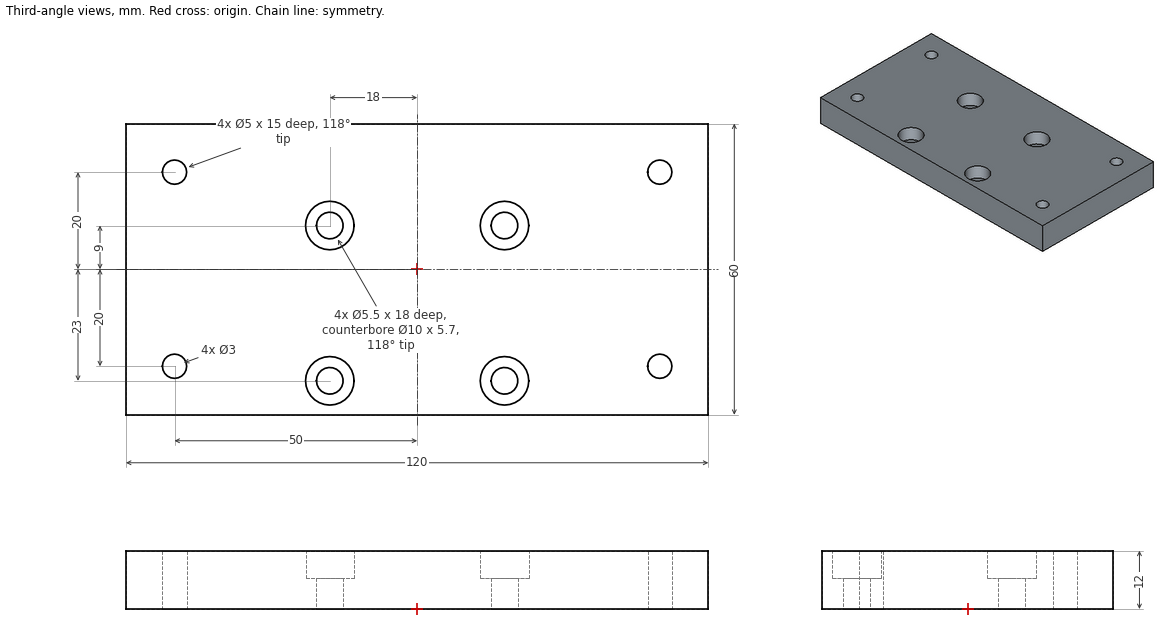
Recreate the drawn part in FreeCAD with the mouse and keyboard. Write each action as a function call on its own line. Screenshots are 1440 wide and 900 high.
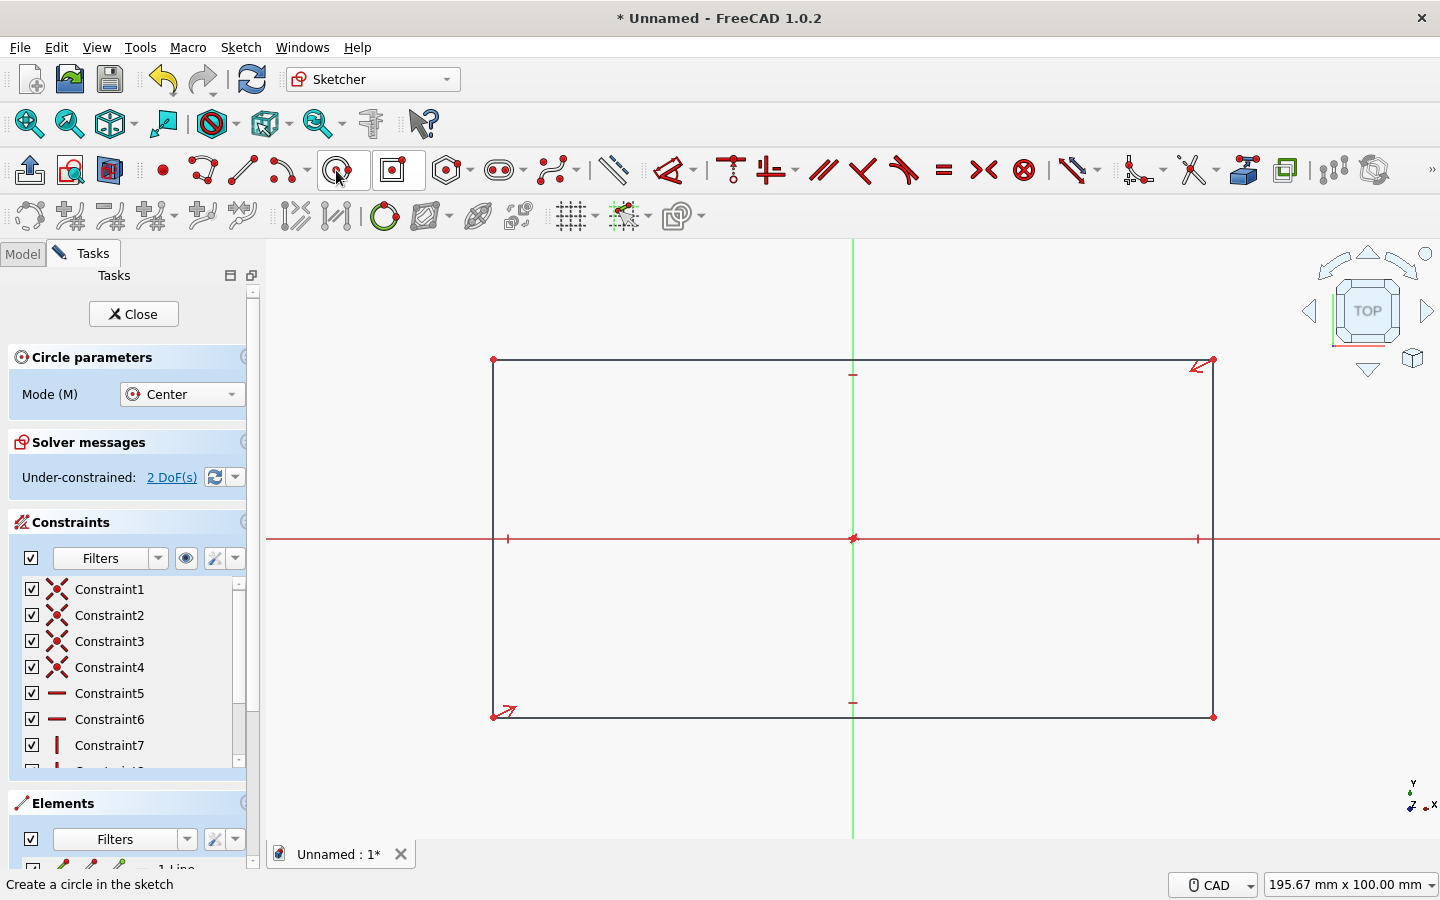
scroll(553, 659, up, 5)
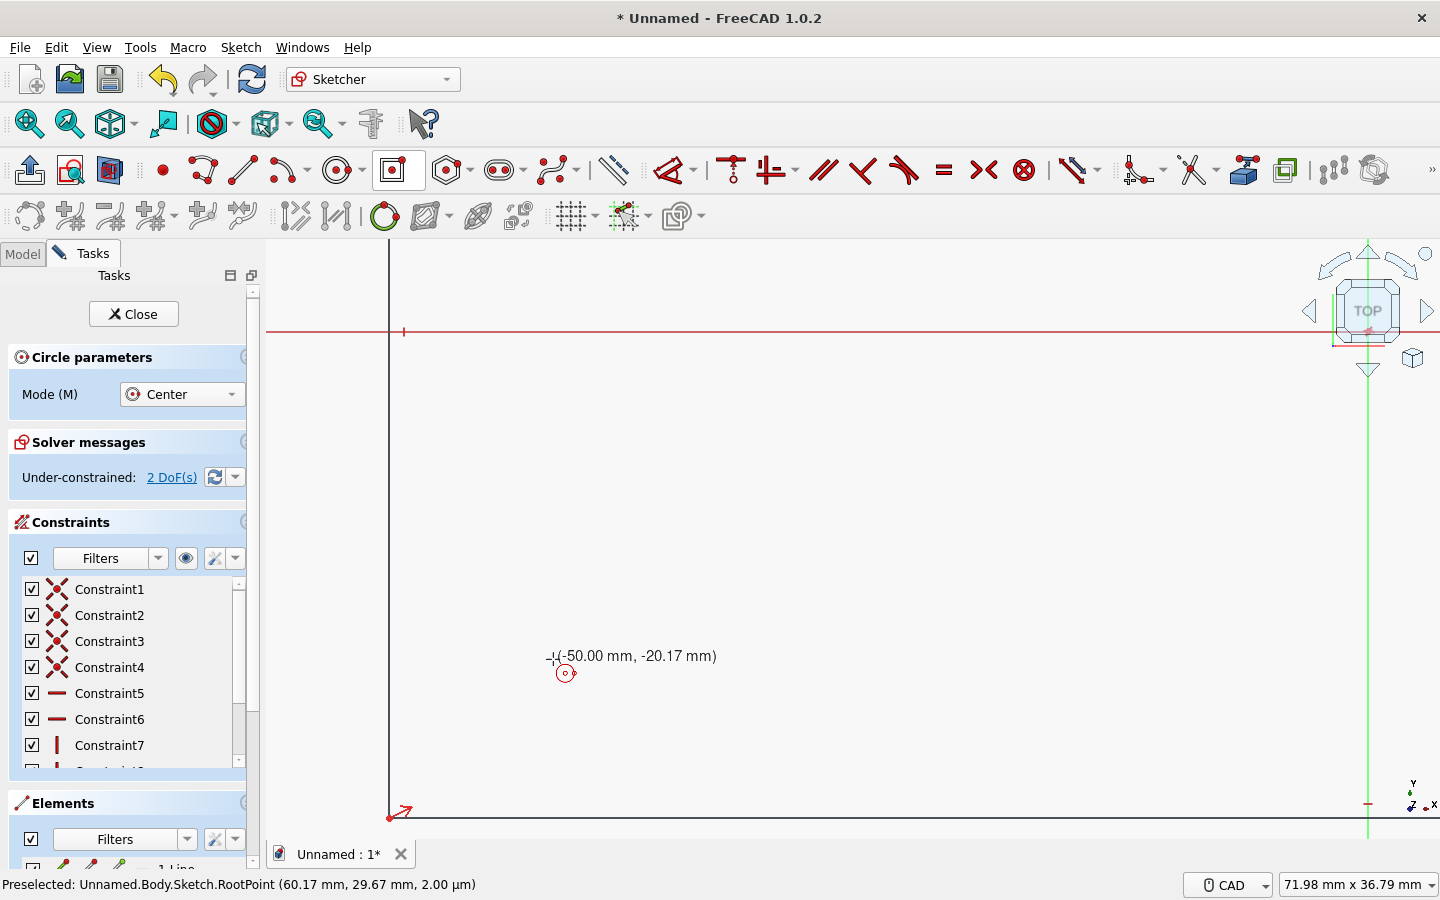
click(553, 658)
click(570, 640)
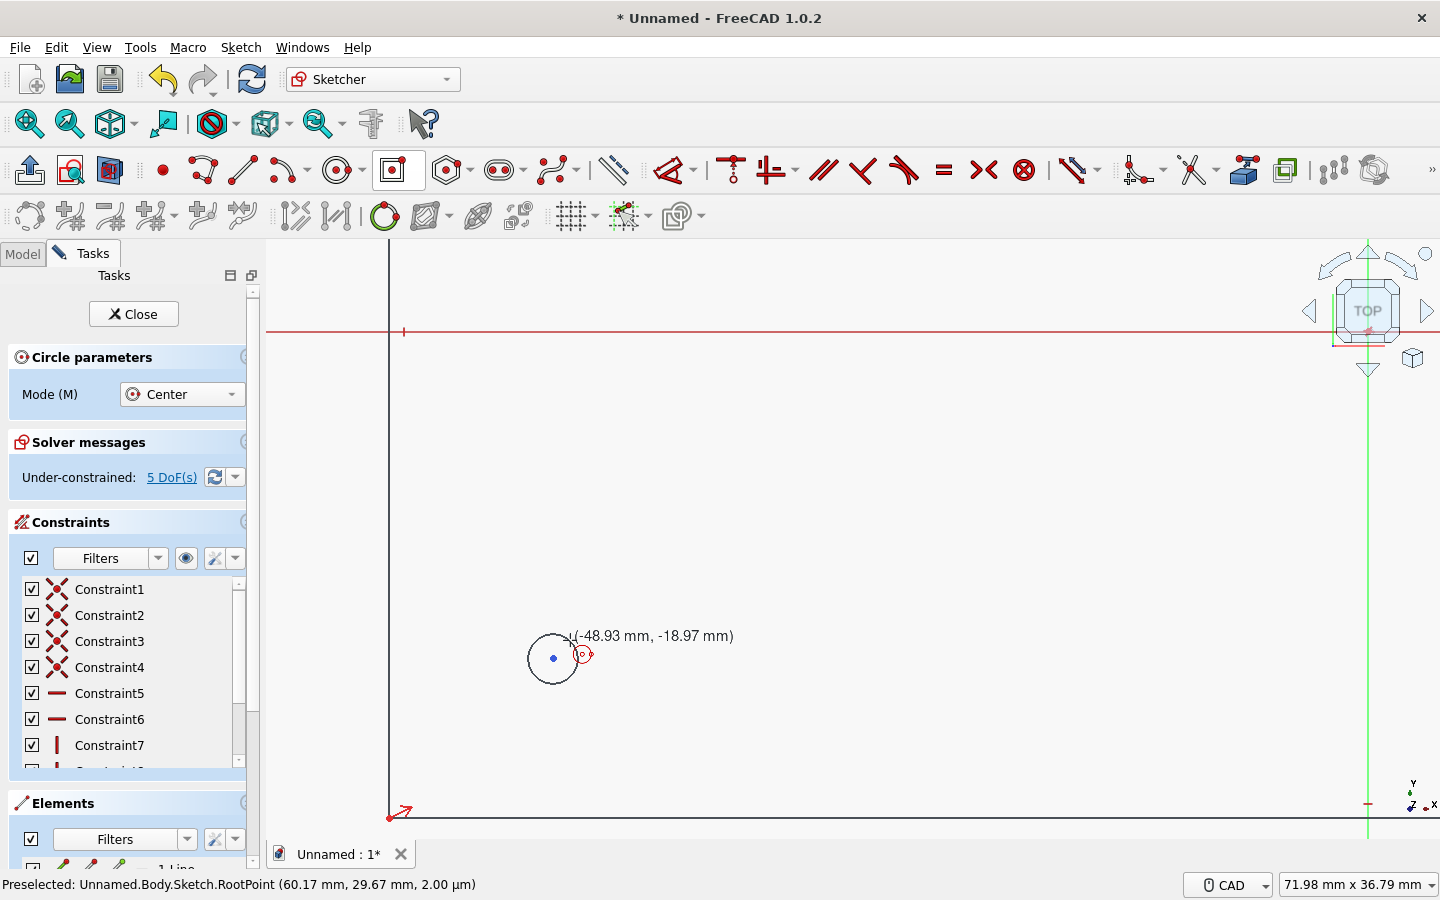
scroll(445, 660, down, 5)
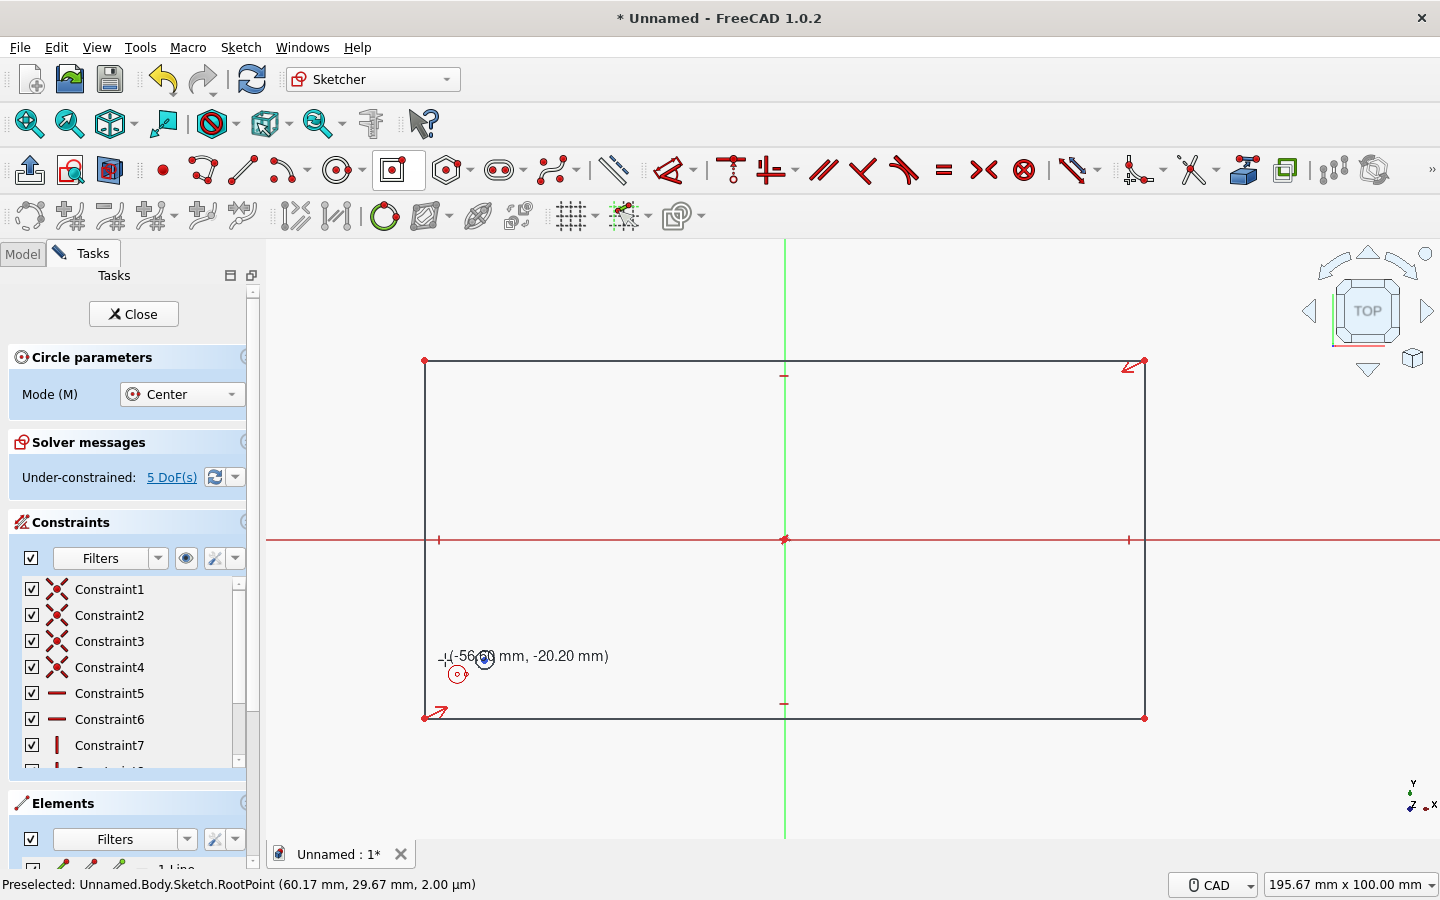
scroll(1085, 660, up, 5)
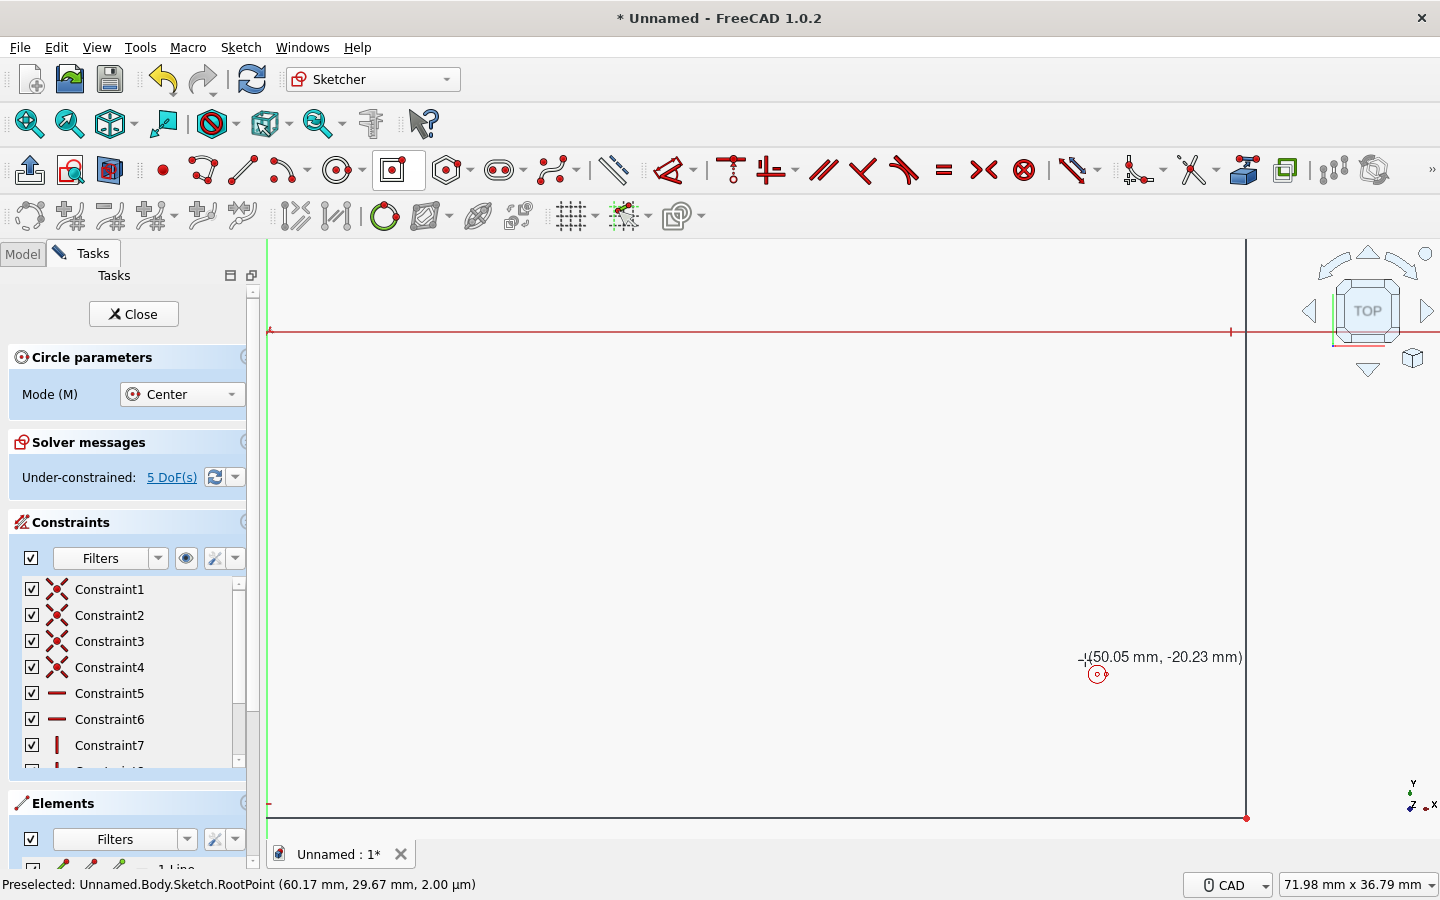
click(1083, 658)
click(1100, 640)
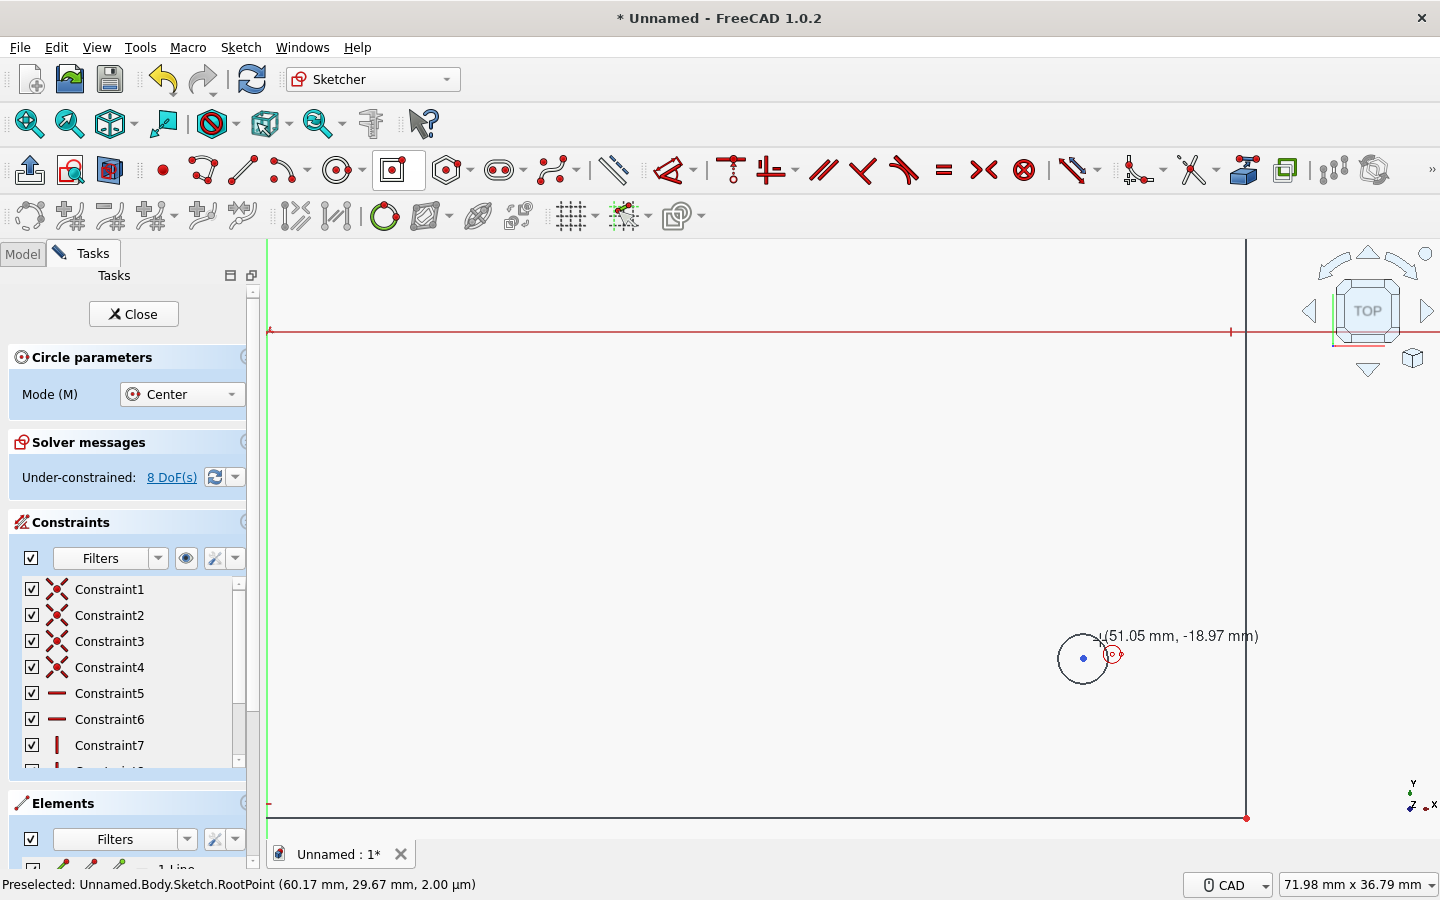
scroll(1085, 660, down, 5)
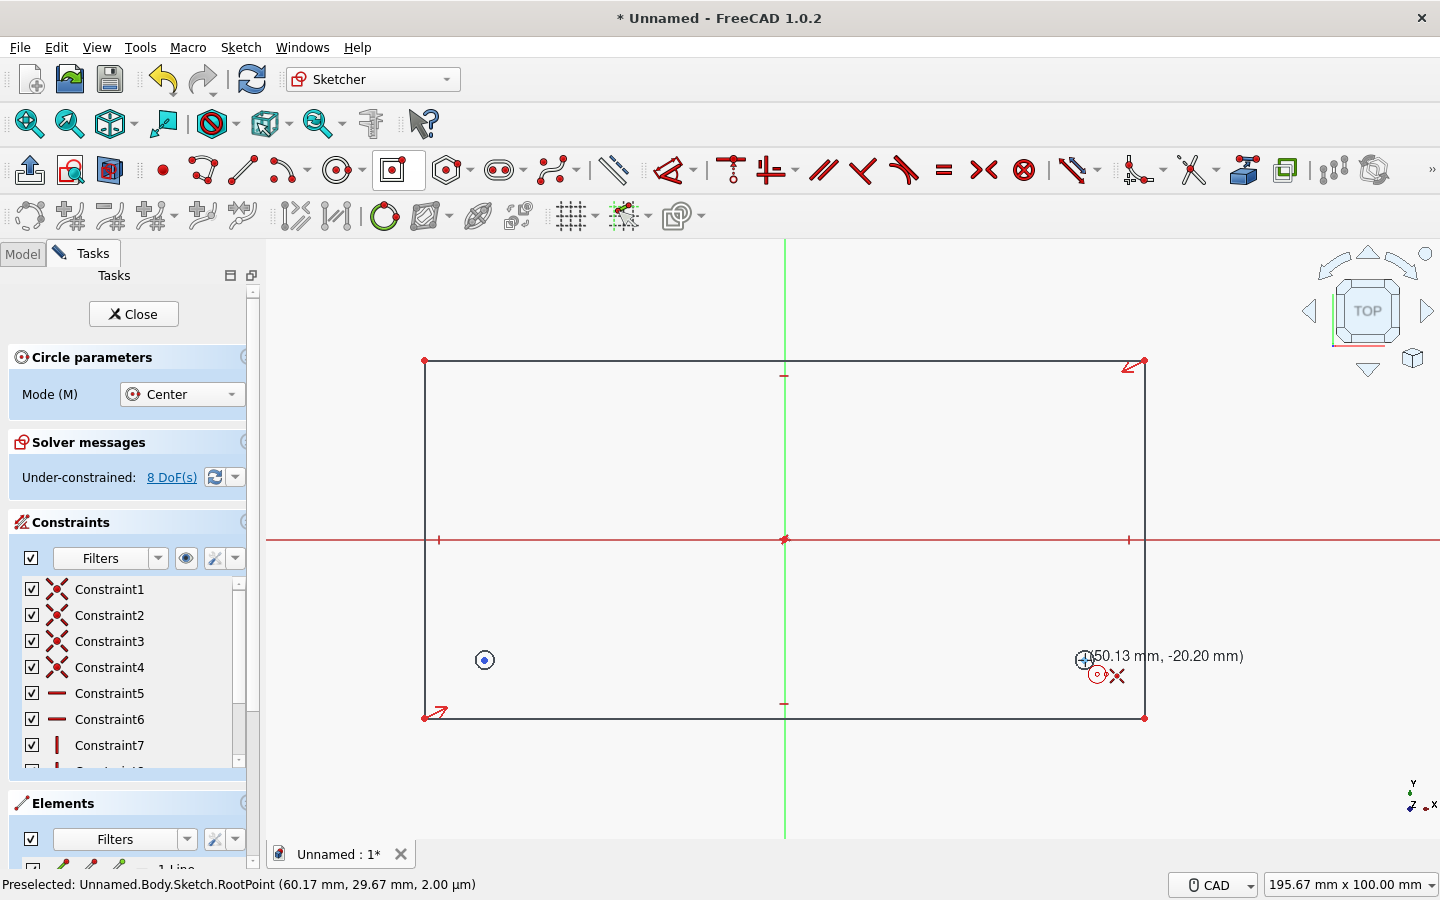
scroll(485, 420, up, 5)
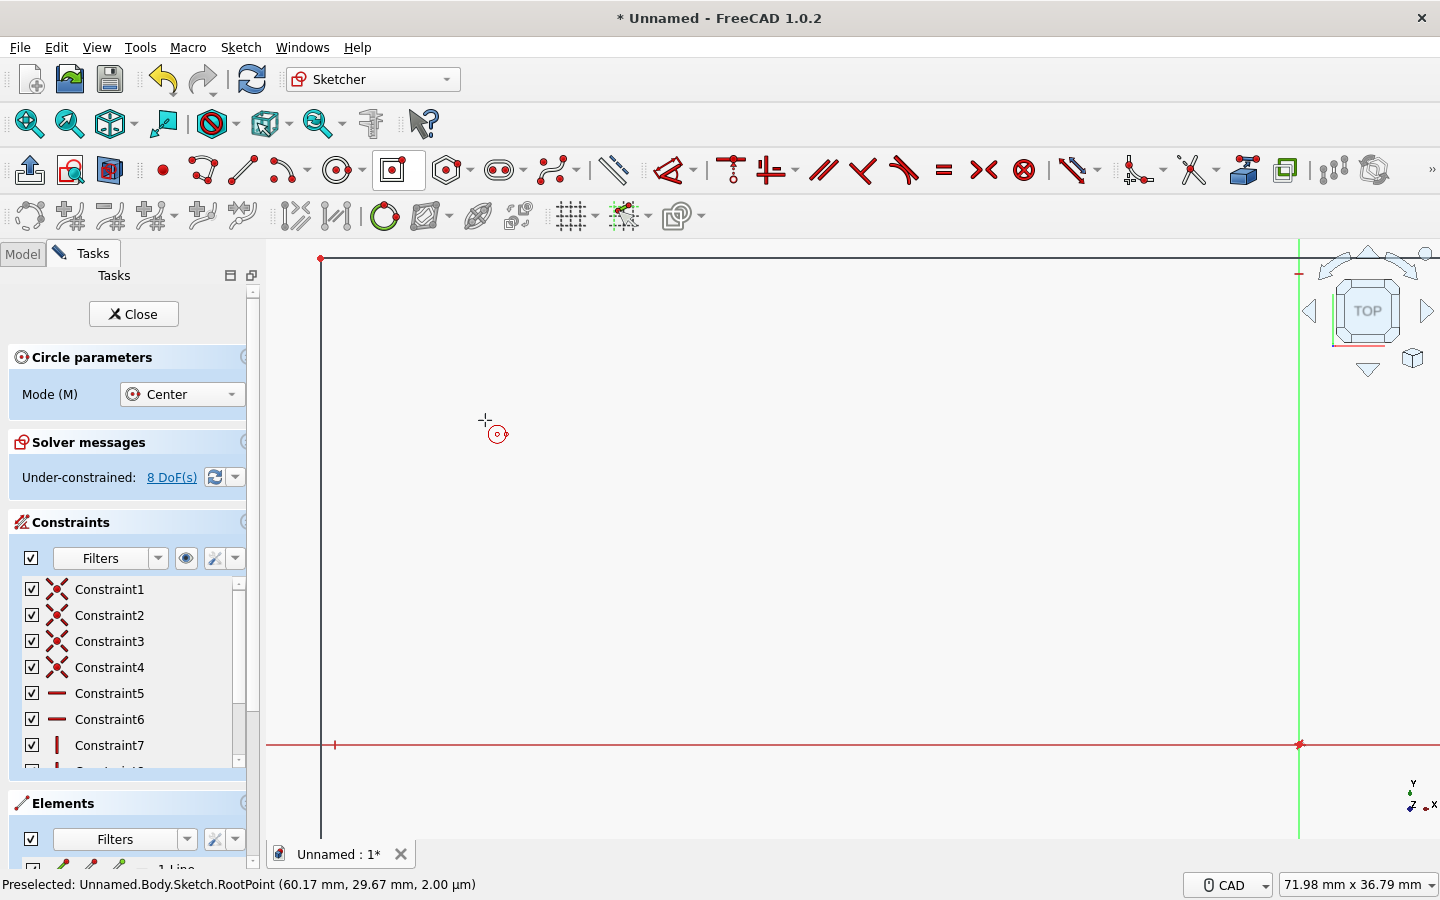
click(484, 418)
click(501, 401)